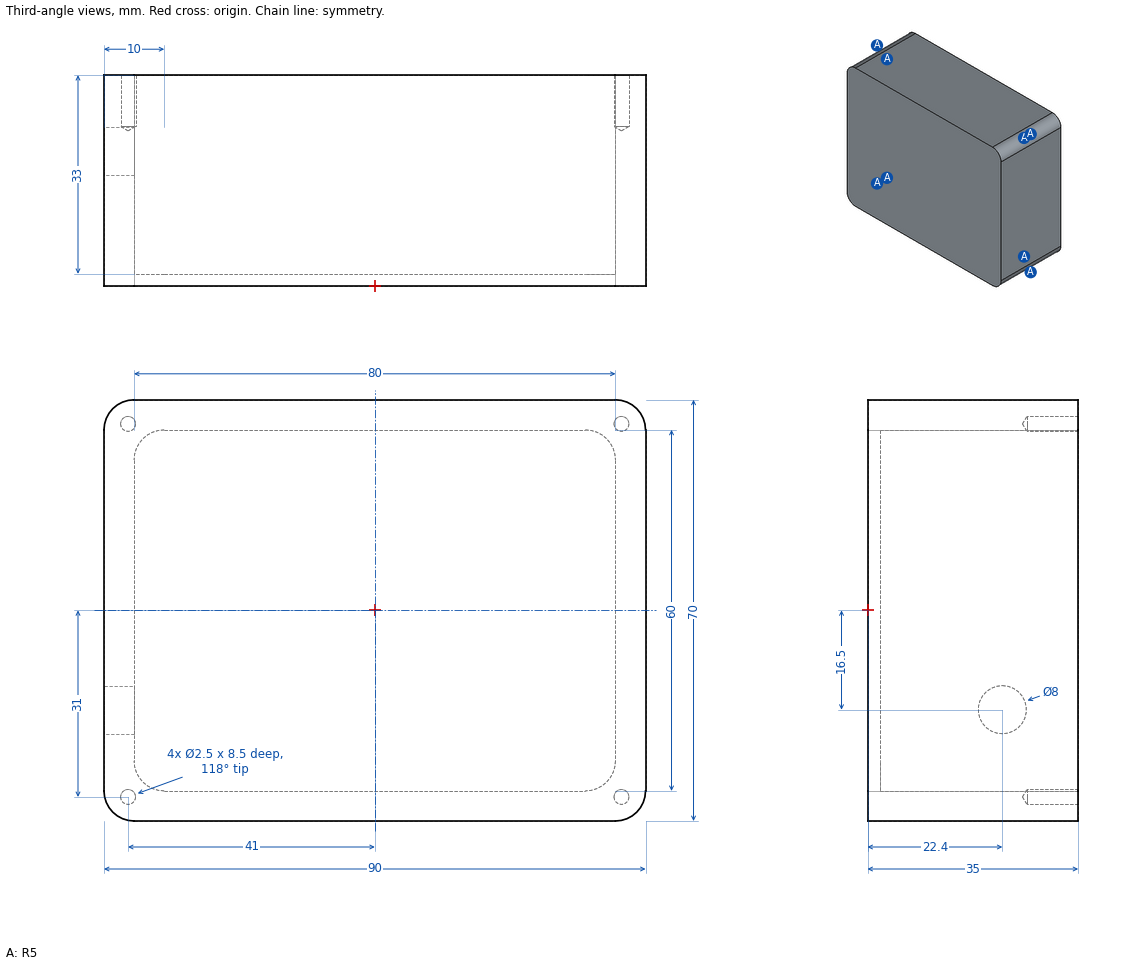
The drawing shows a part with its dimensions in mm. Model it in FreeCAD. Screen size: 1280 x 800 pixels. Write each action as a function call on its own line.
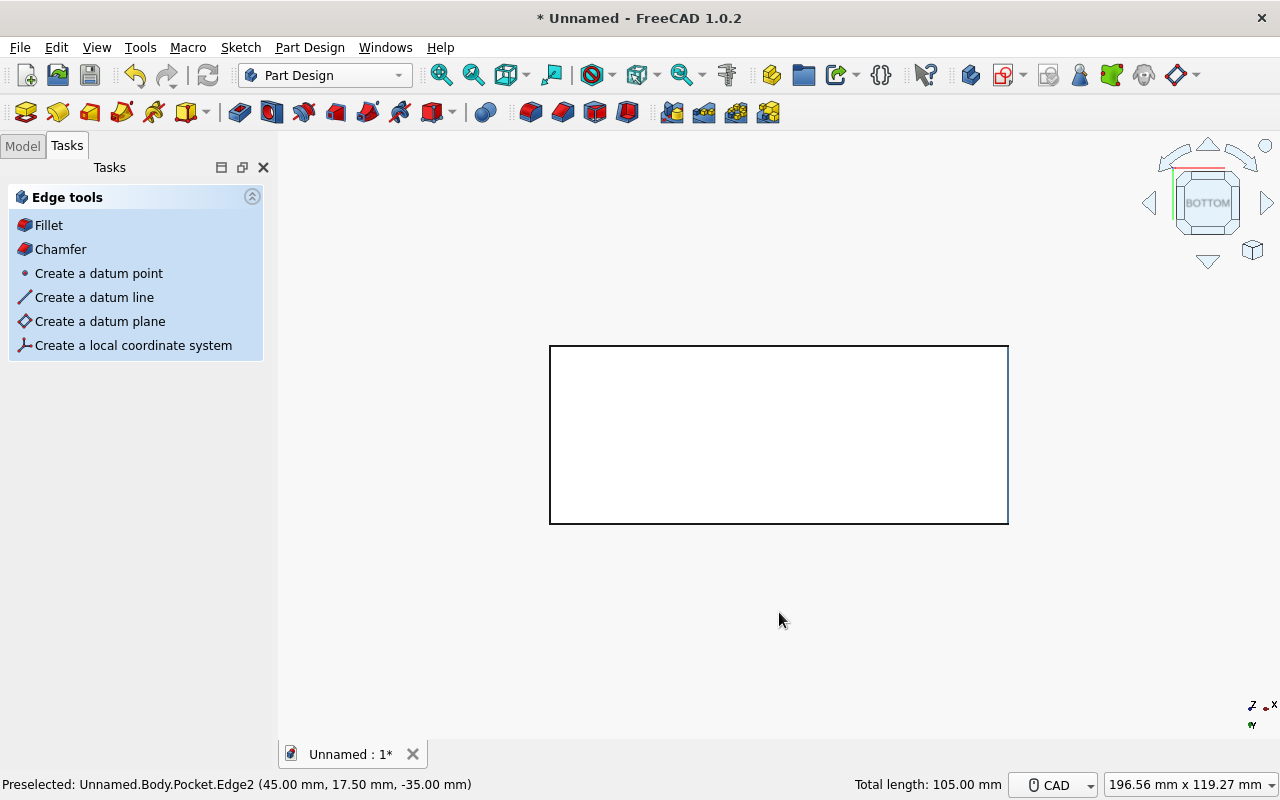
click(550, 434, ctrl)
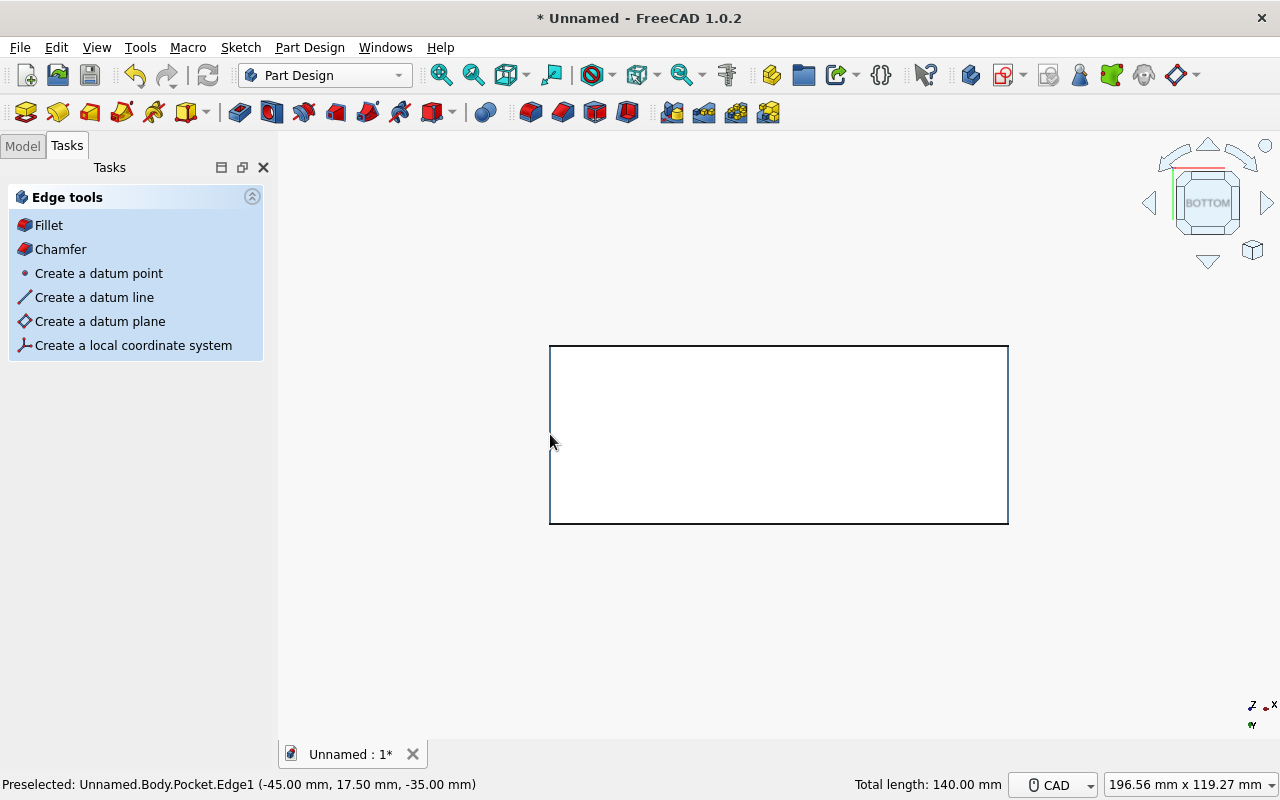
key(4)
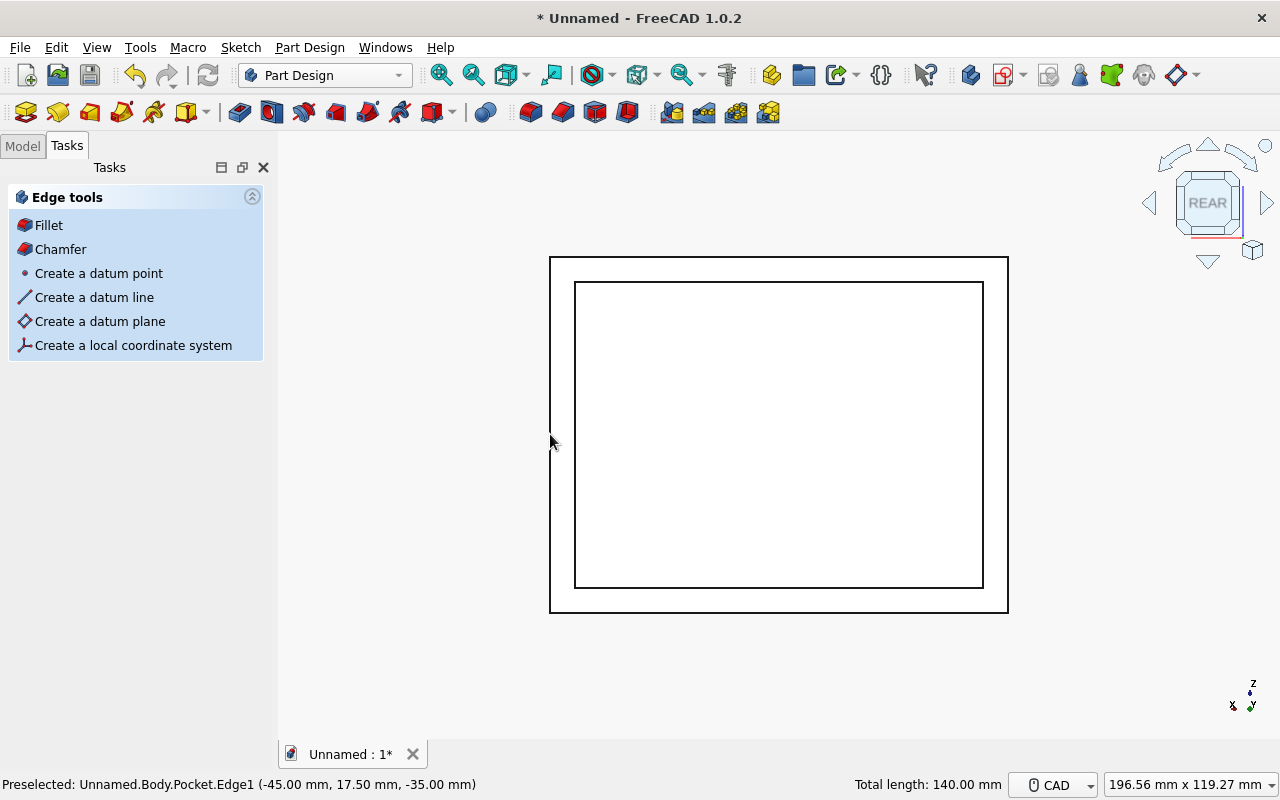
key(6)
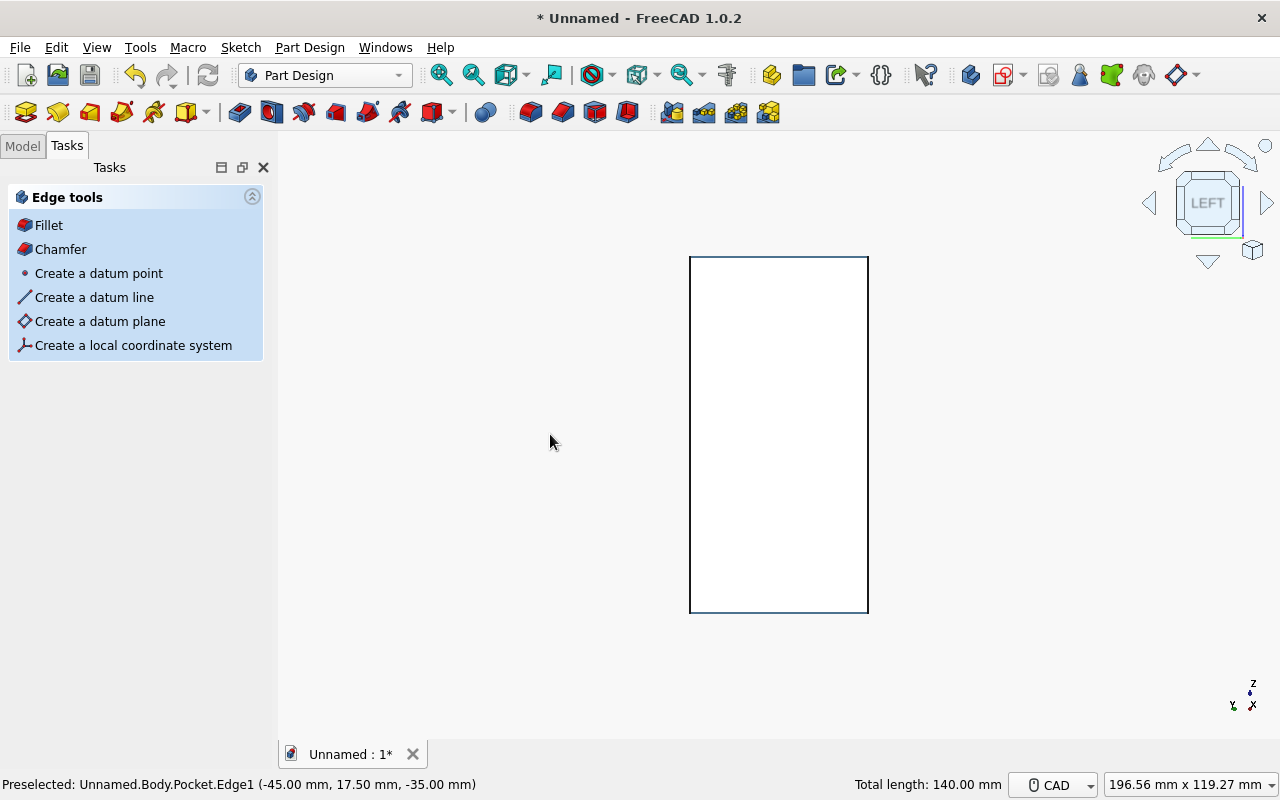
key(v)
key(3)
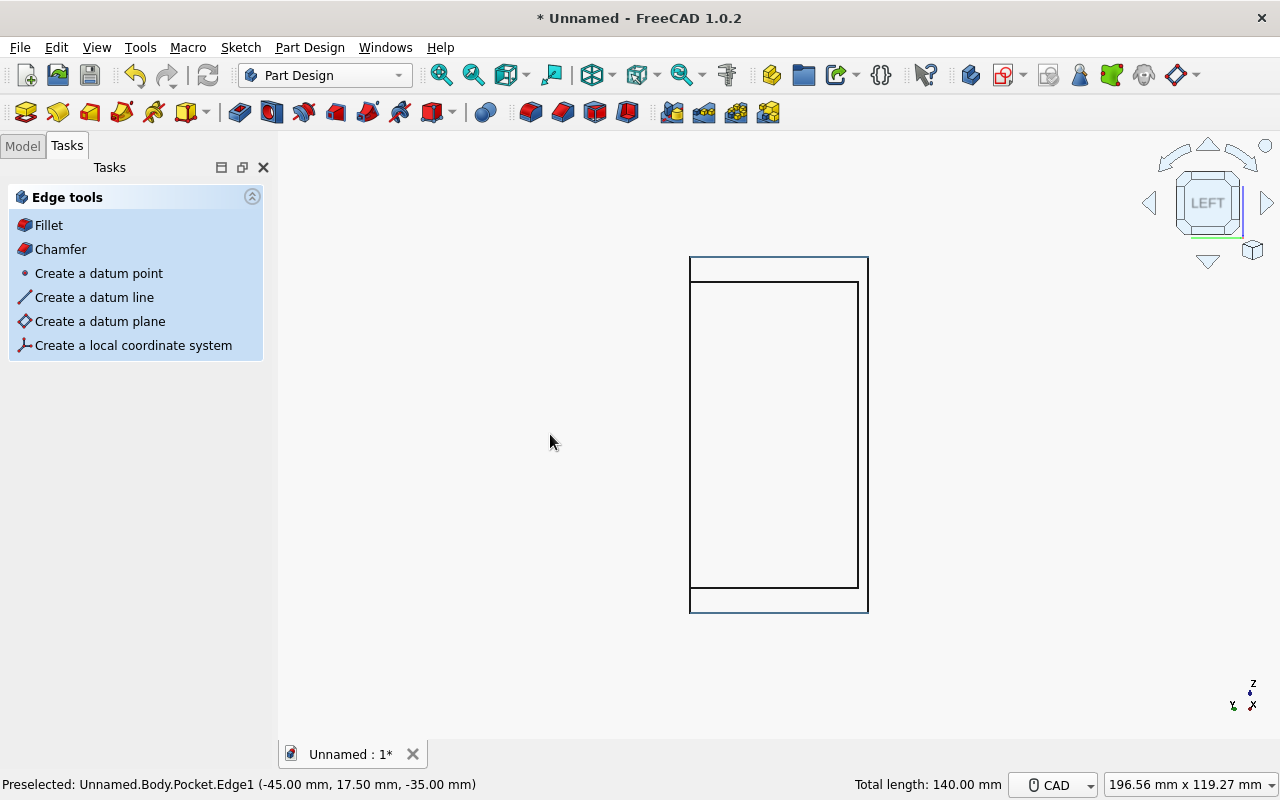
key(0)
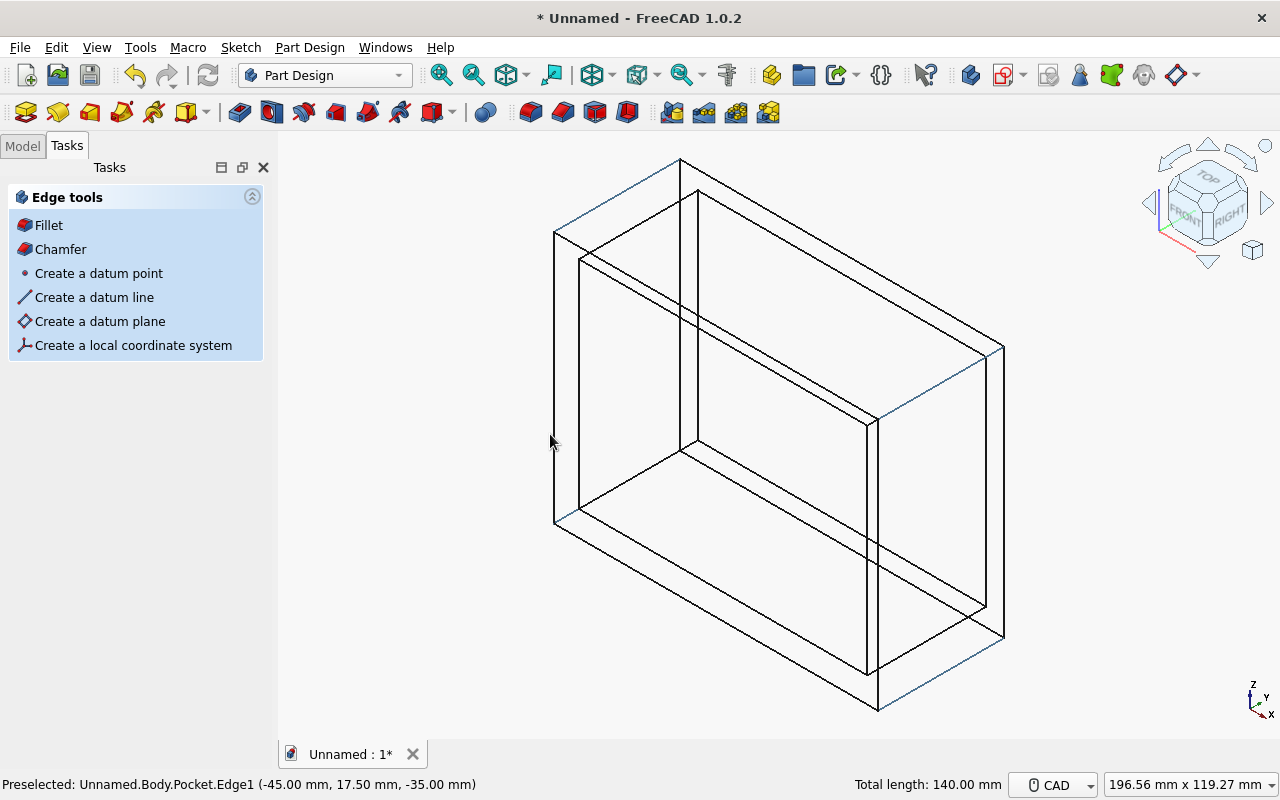
click(927, 640, ctrl)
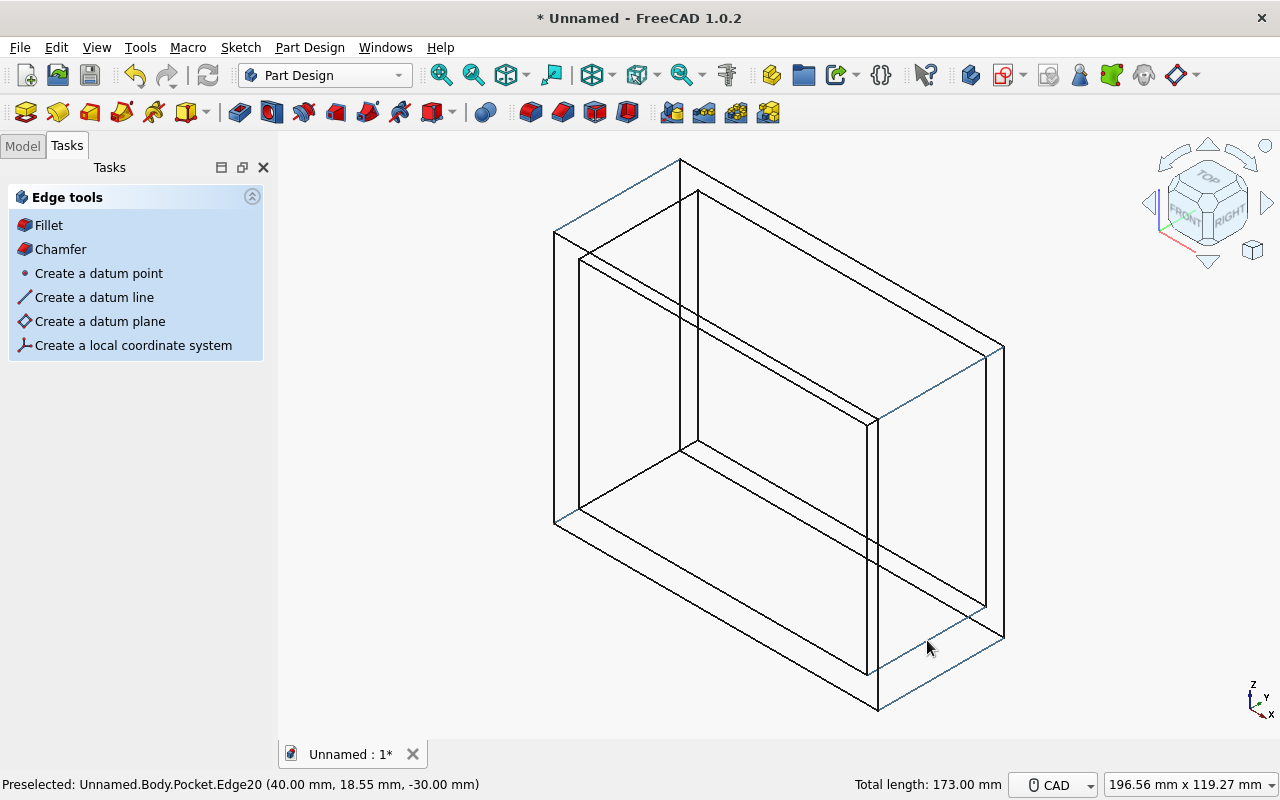
click(638, 224, ctrl)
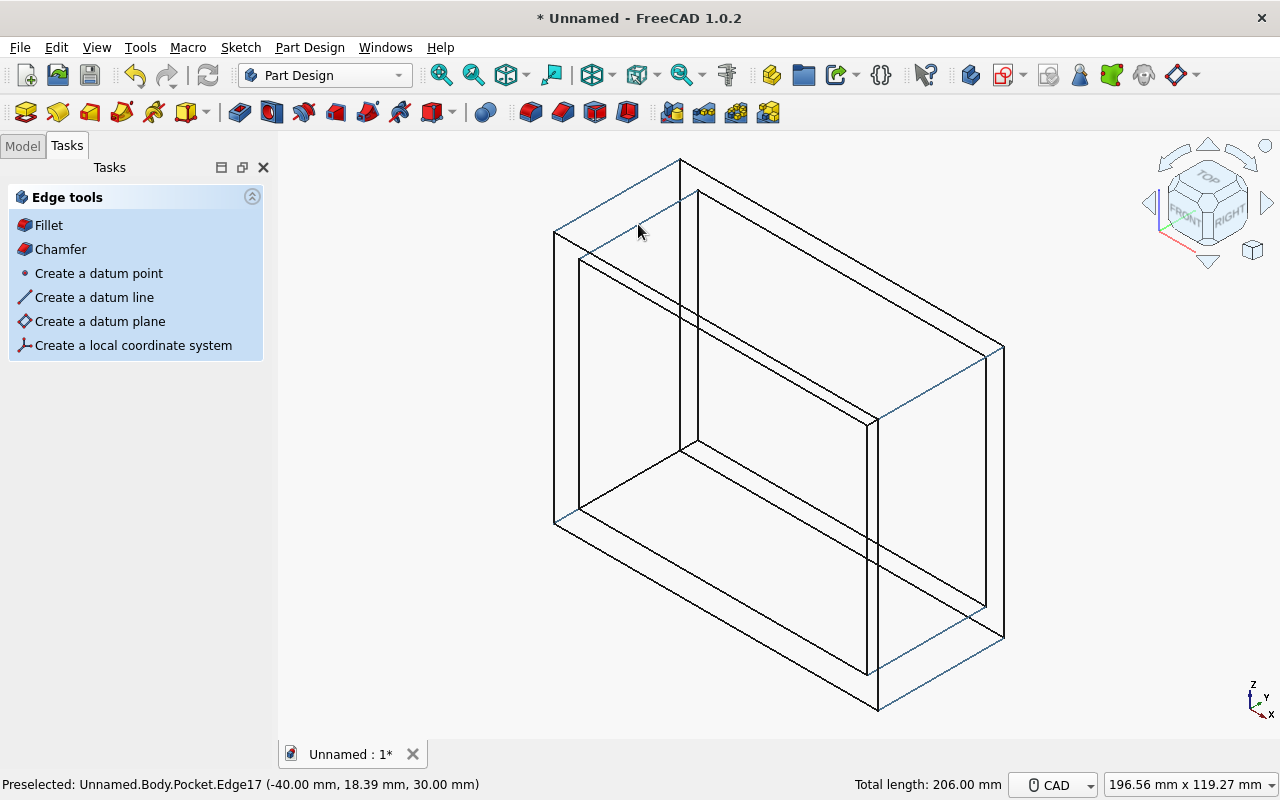
click(638, 474, ctrl)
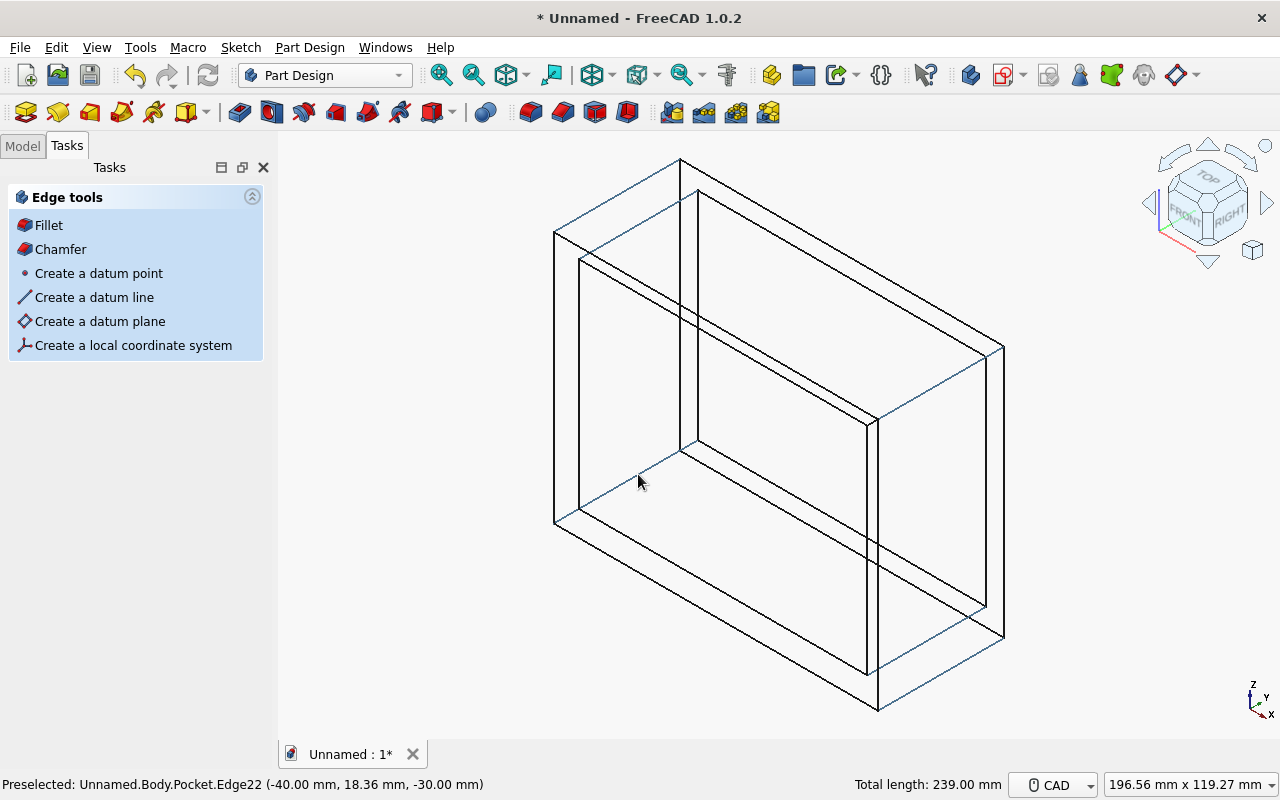
scroll(927, 390, up, 6)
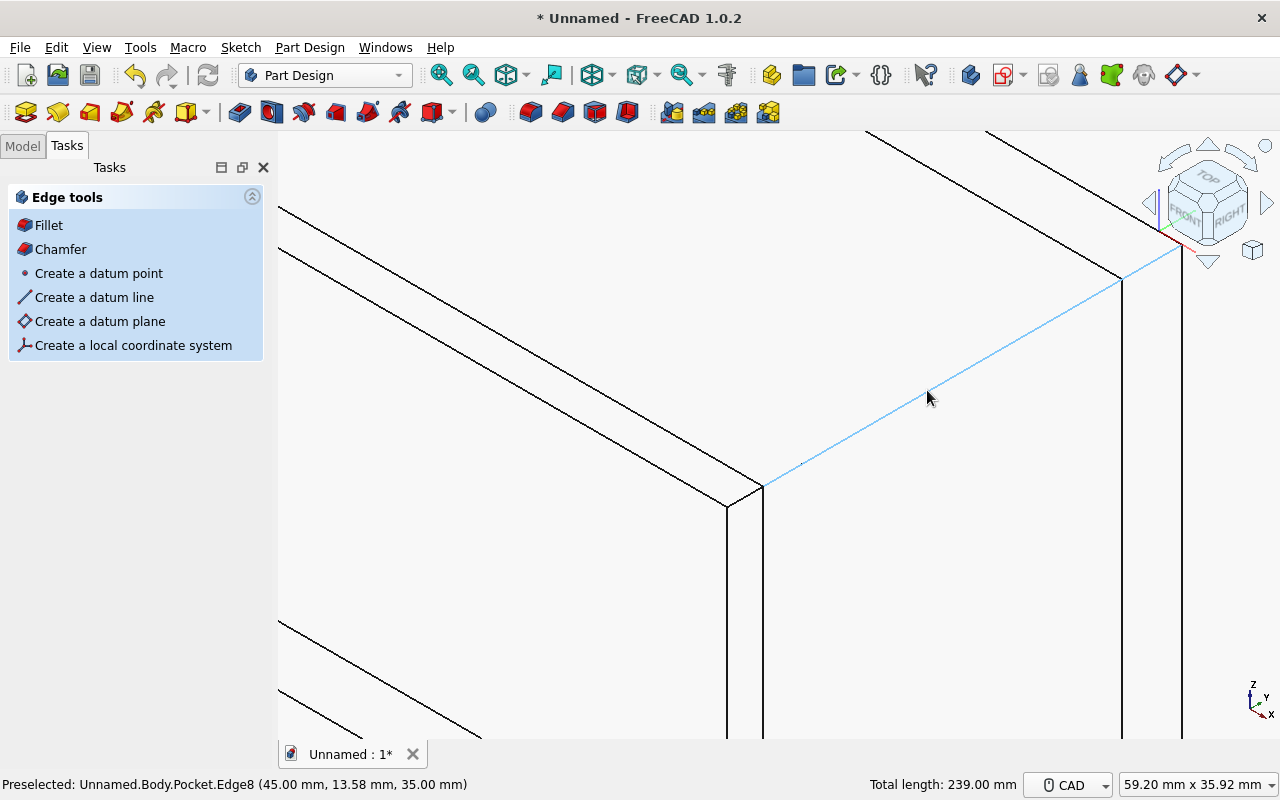
key(v)
key(f)